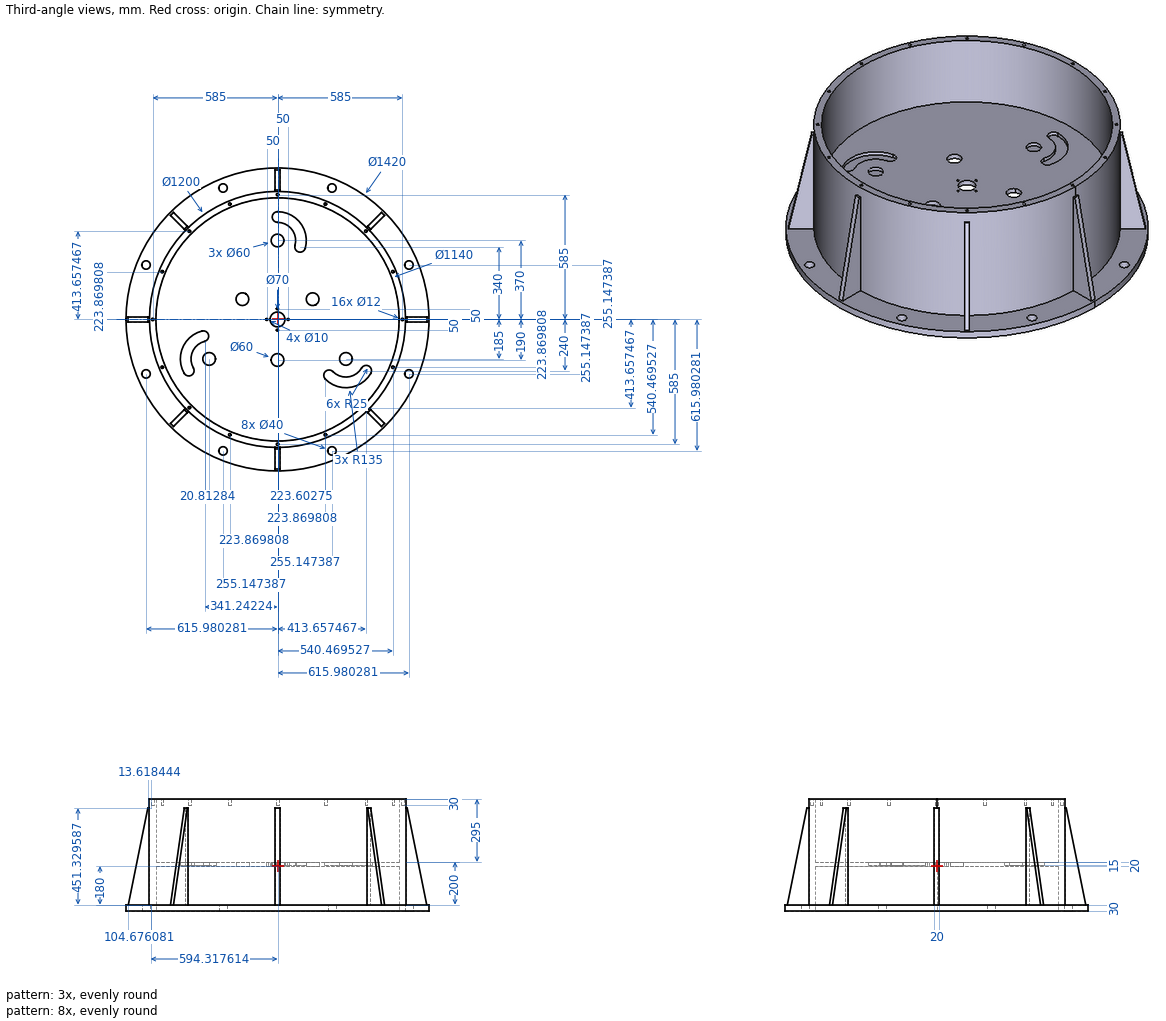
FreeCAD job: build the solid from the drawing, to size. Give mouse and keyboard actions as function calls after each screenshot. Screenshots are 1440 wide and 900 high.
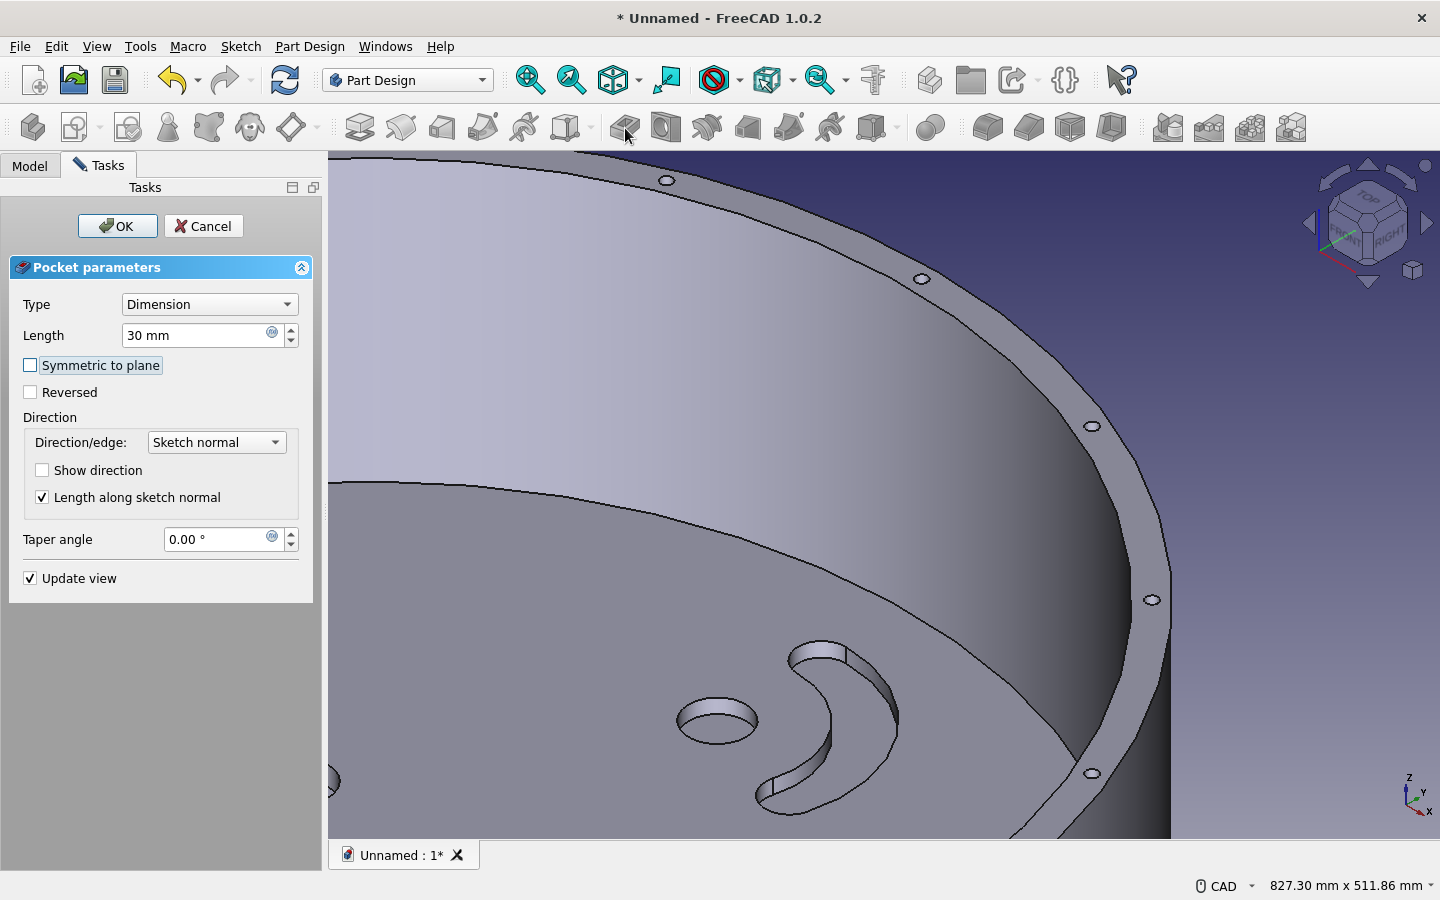
click(118, 226)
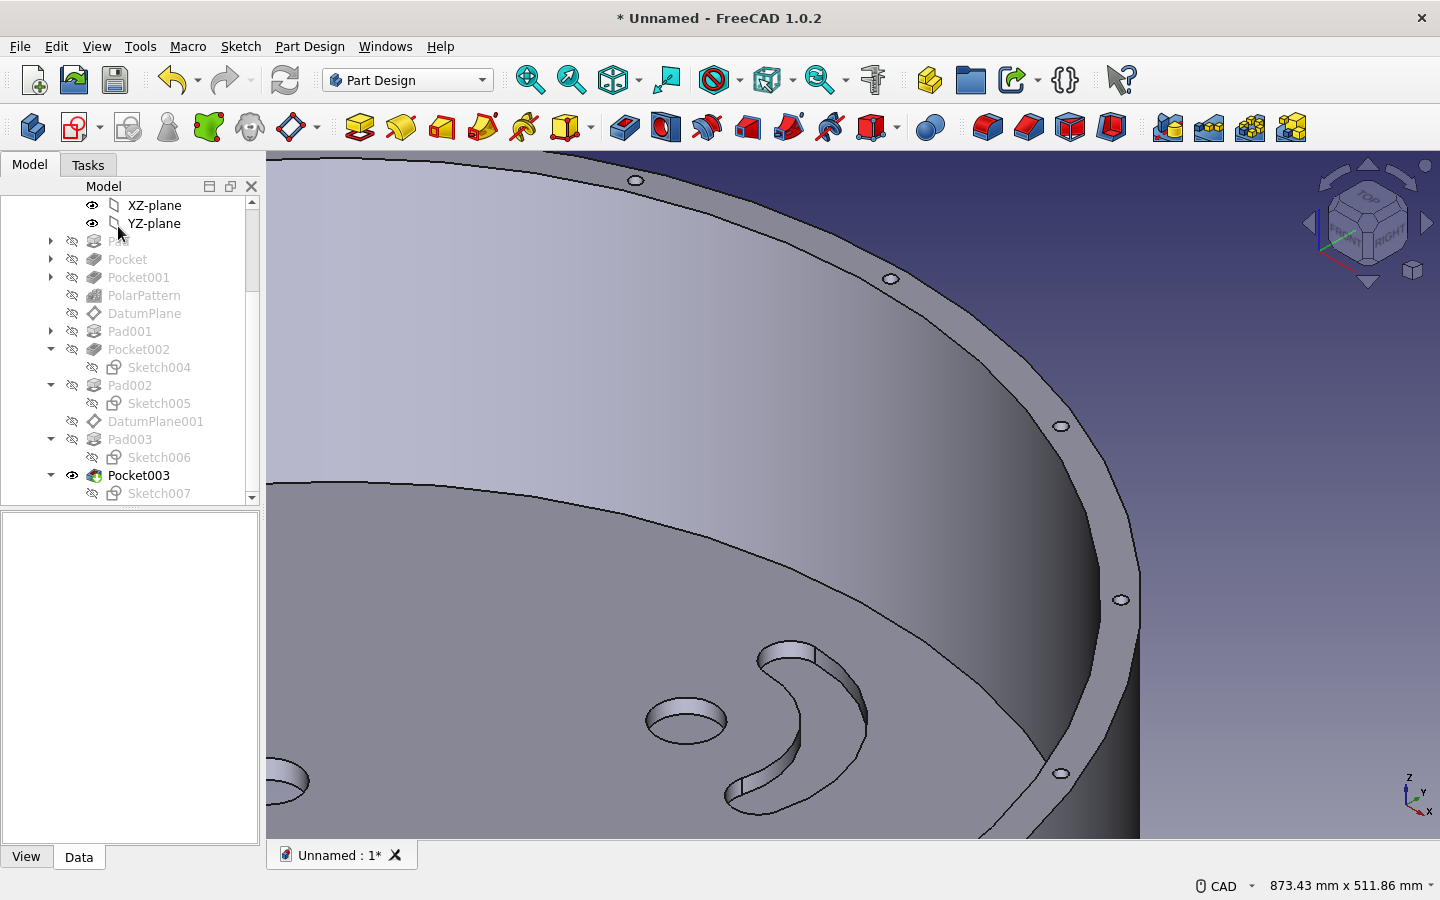
key(v)
key(f)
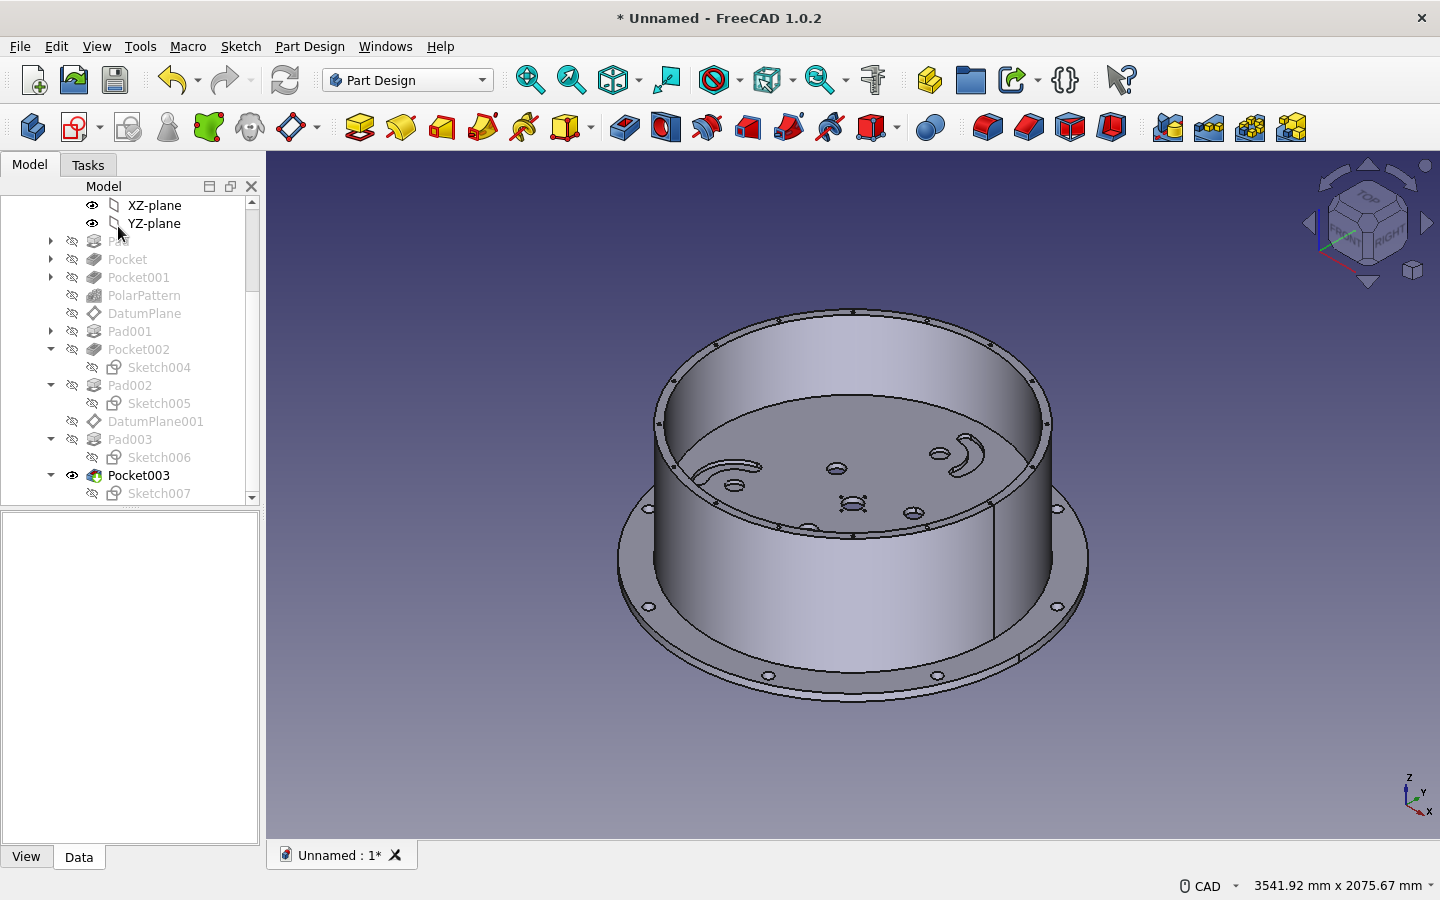
click(74, 128)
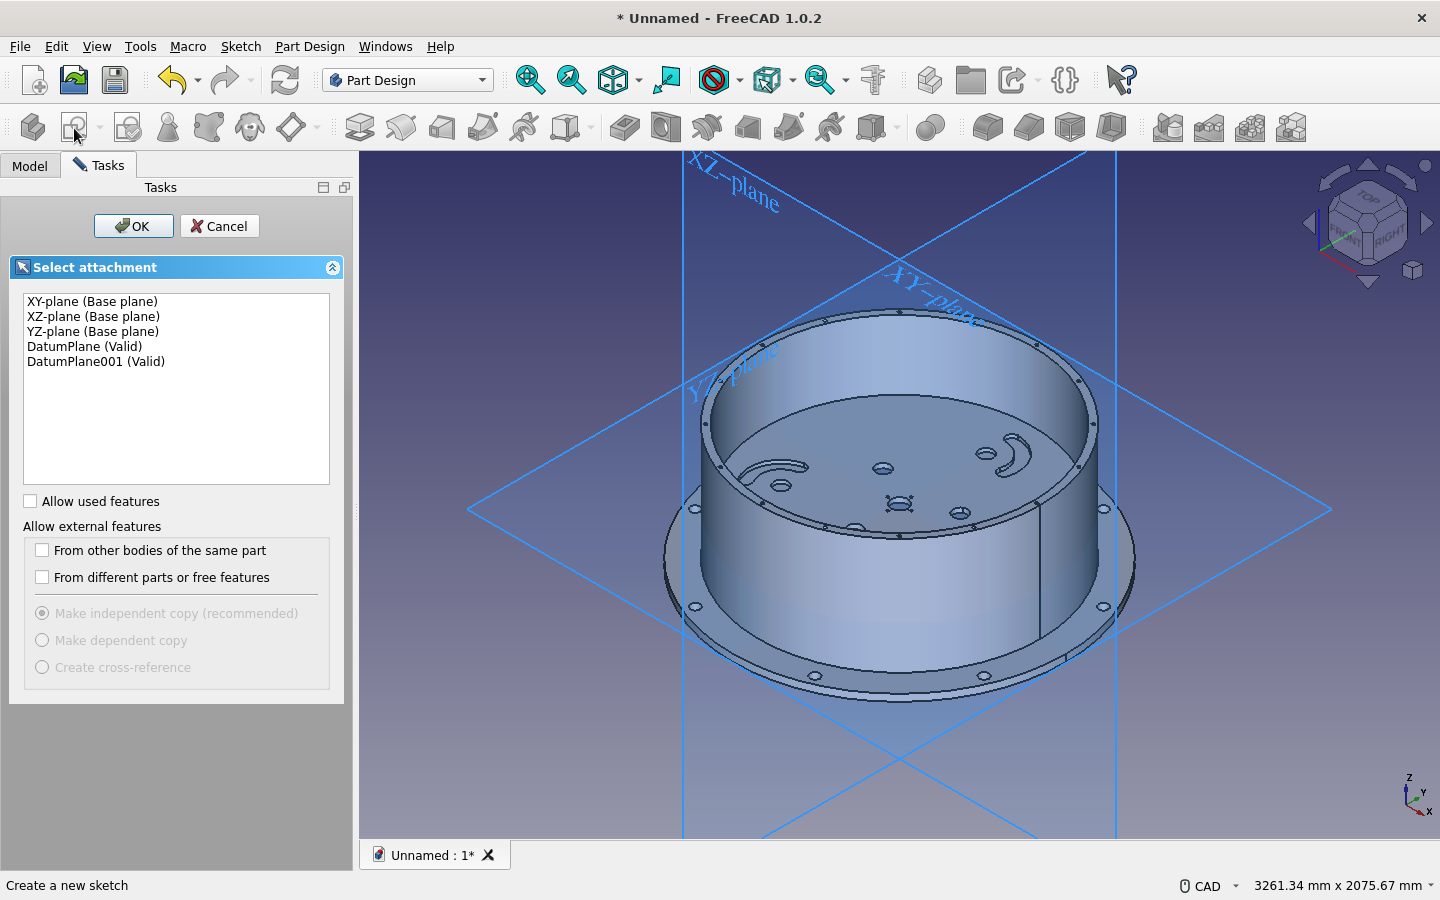
click(84, 316)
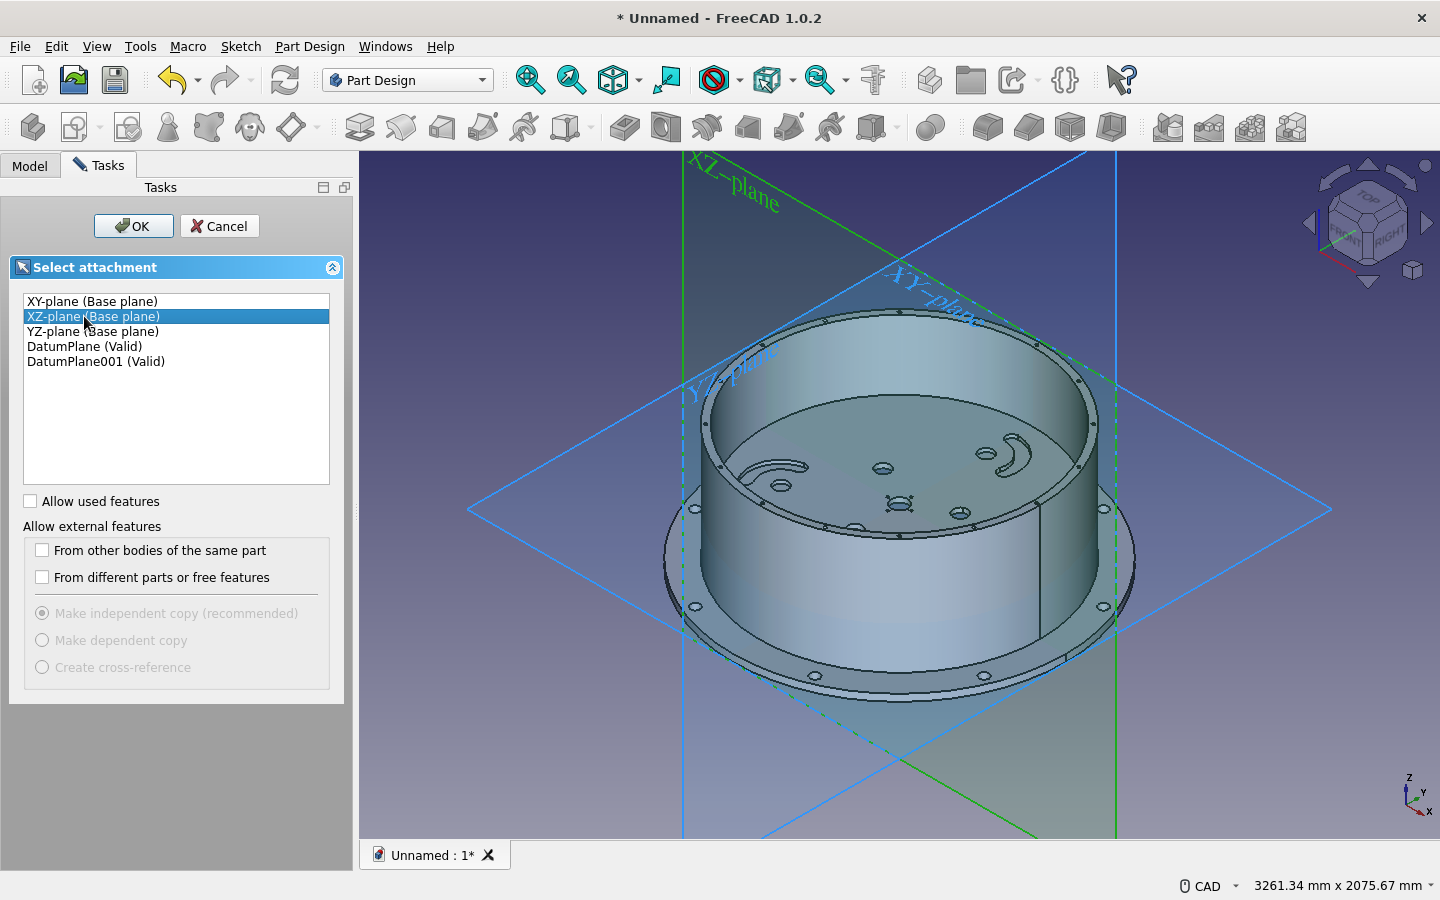
click(134, 226)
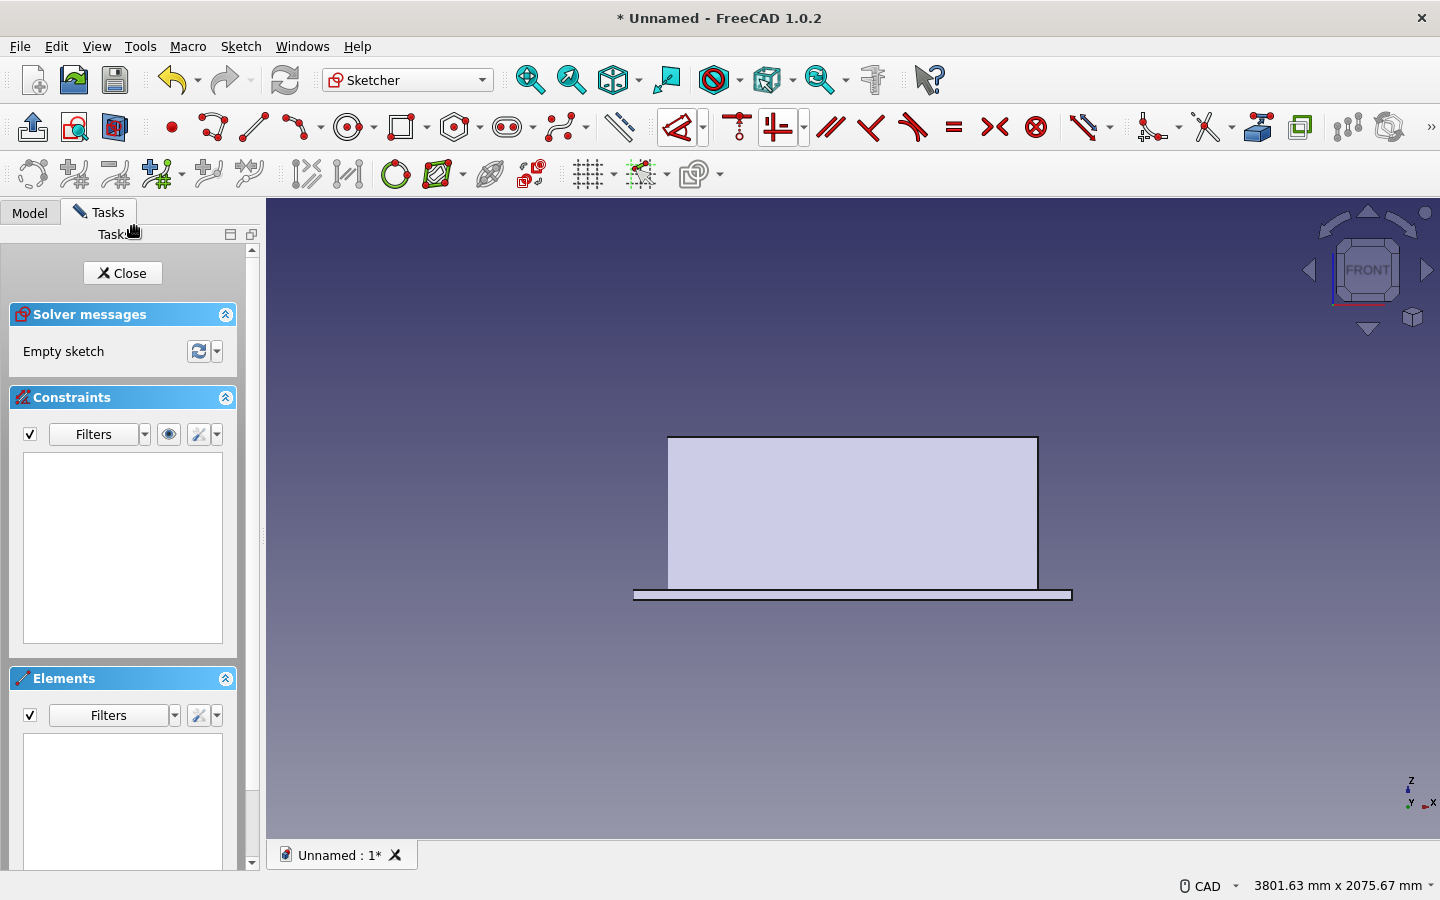
click(115, 128)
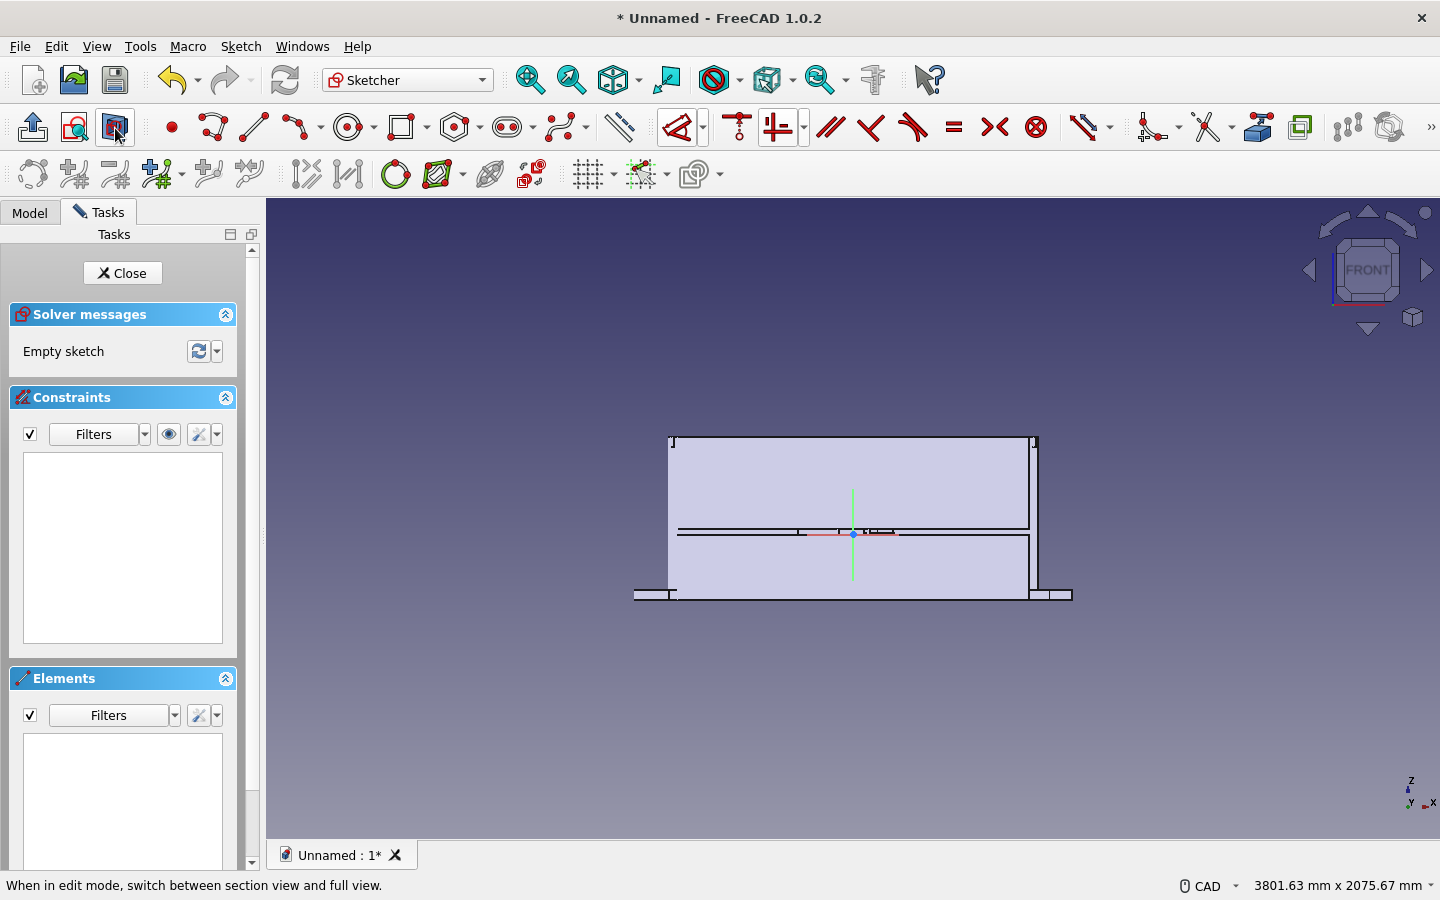
scroll(722, 522, up, 5)